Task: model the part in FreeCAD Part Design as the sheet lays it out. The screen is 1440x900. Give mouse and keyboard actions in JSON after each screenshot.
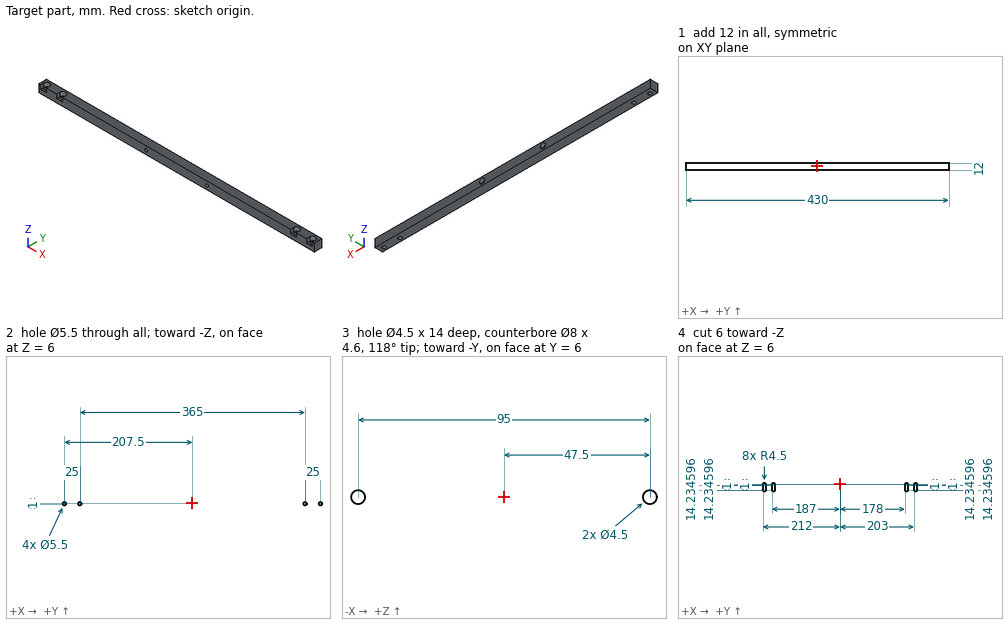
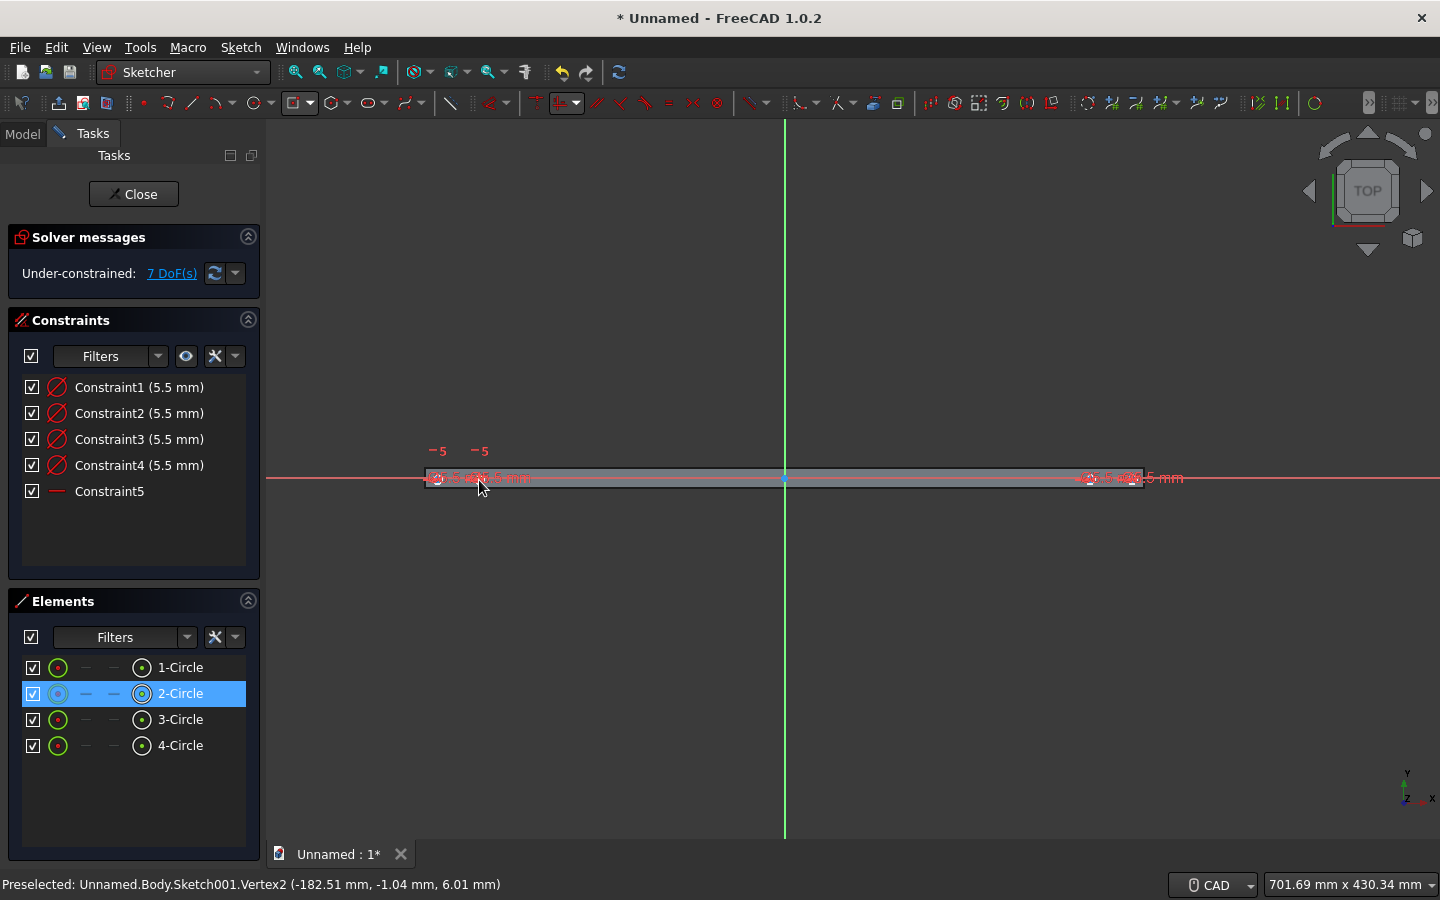
{"action": "left_click", "coordinate": [1090, 480]}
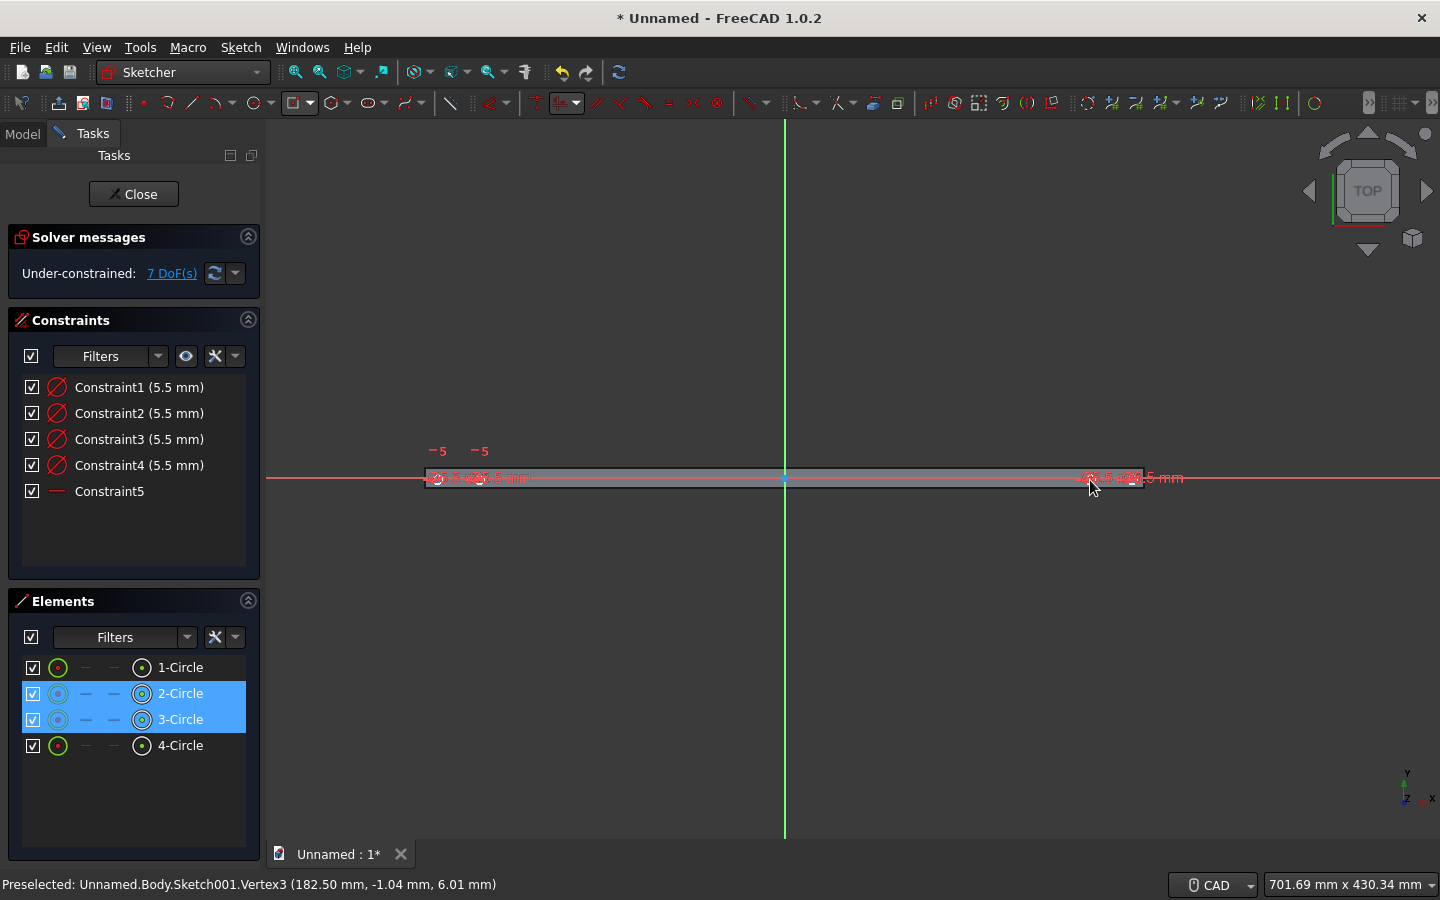
{"action": "left_click", "coordinate": [578, 104]}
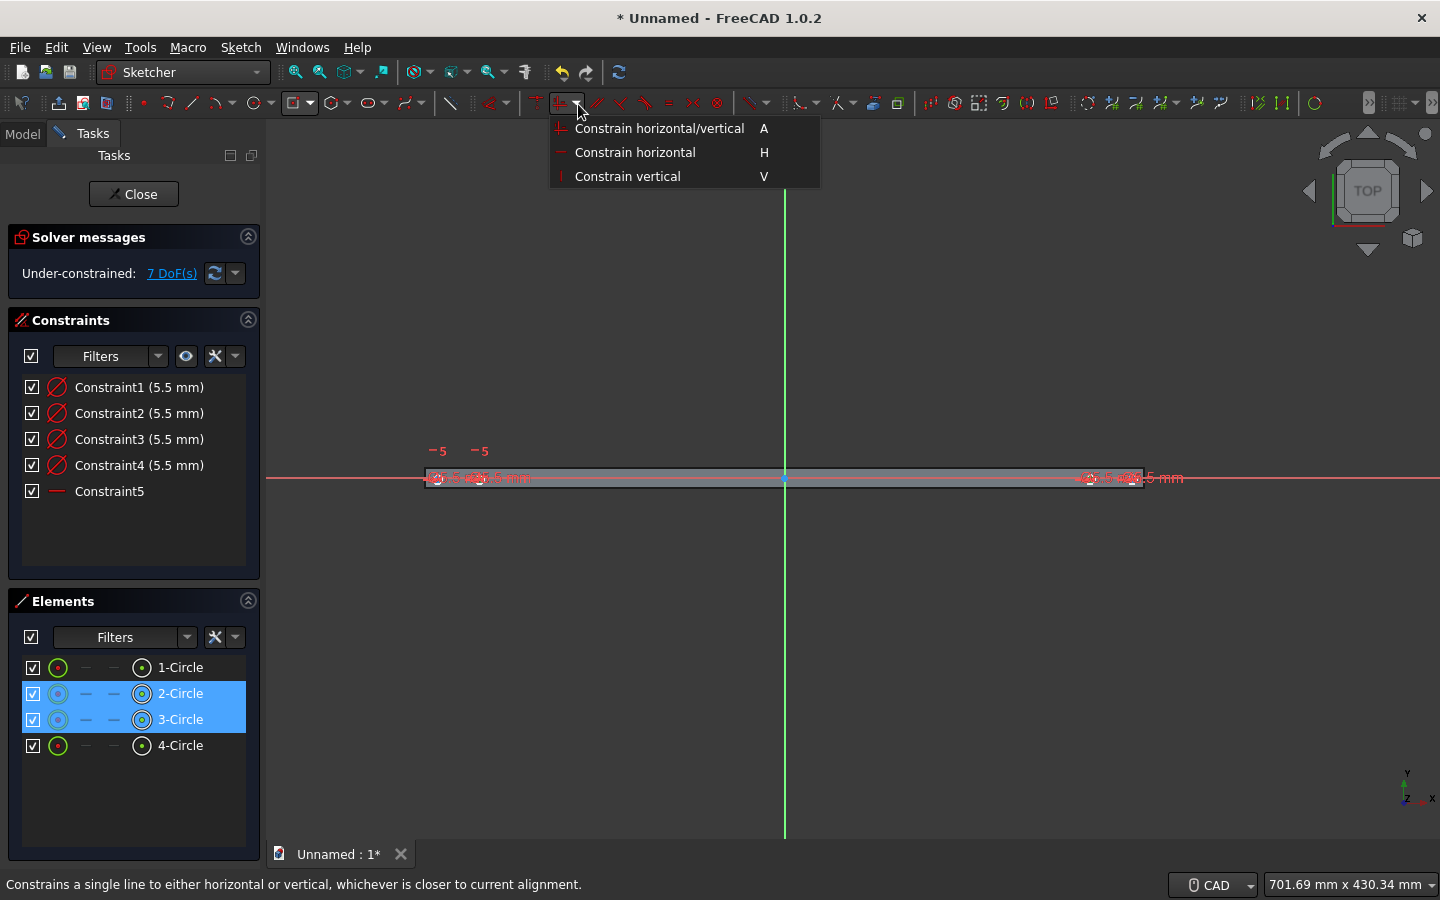
{"action": "left_click", "coordinate": [685, 152]}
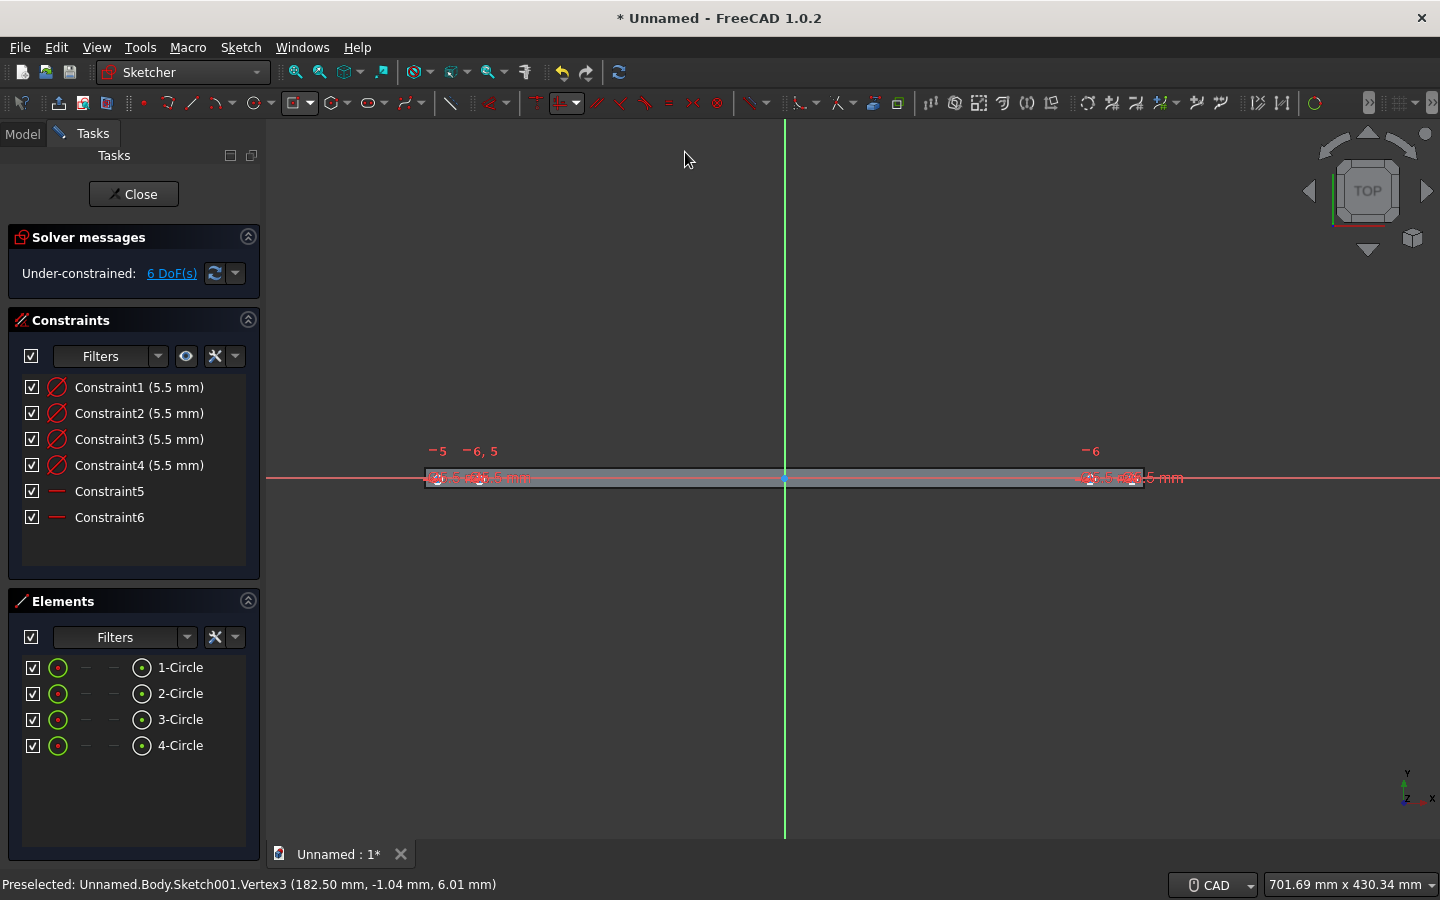
{"action": "left_click", "coordinate": [1090, 480]}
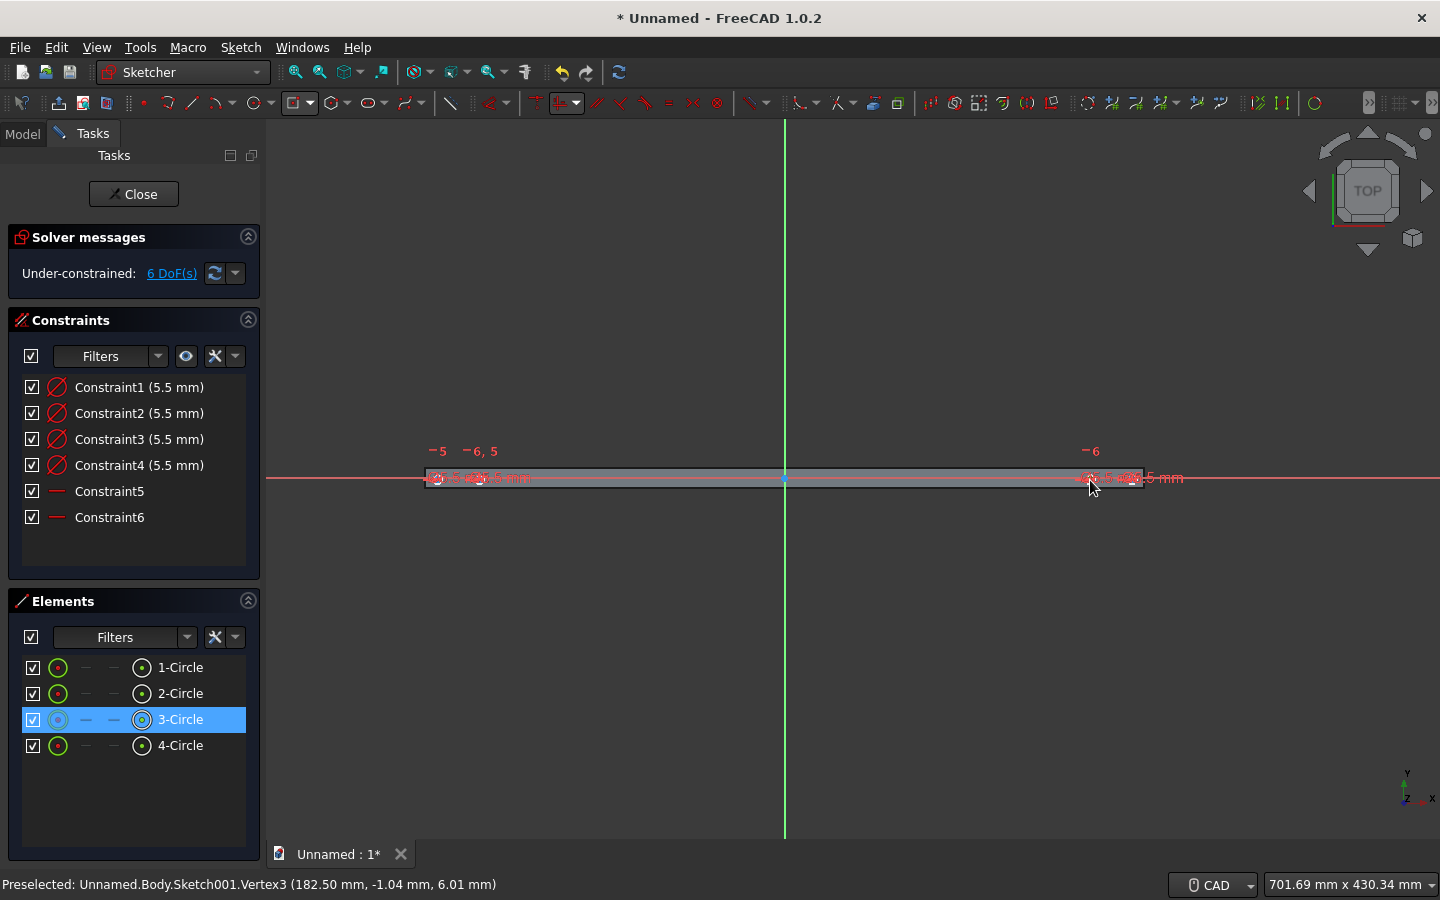
{"action": "left_click", "coordinate": [1132, 480]}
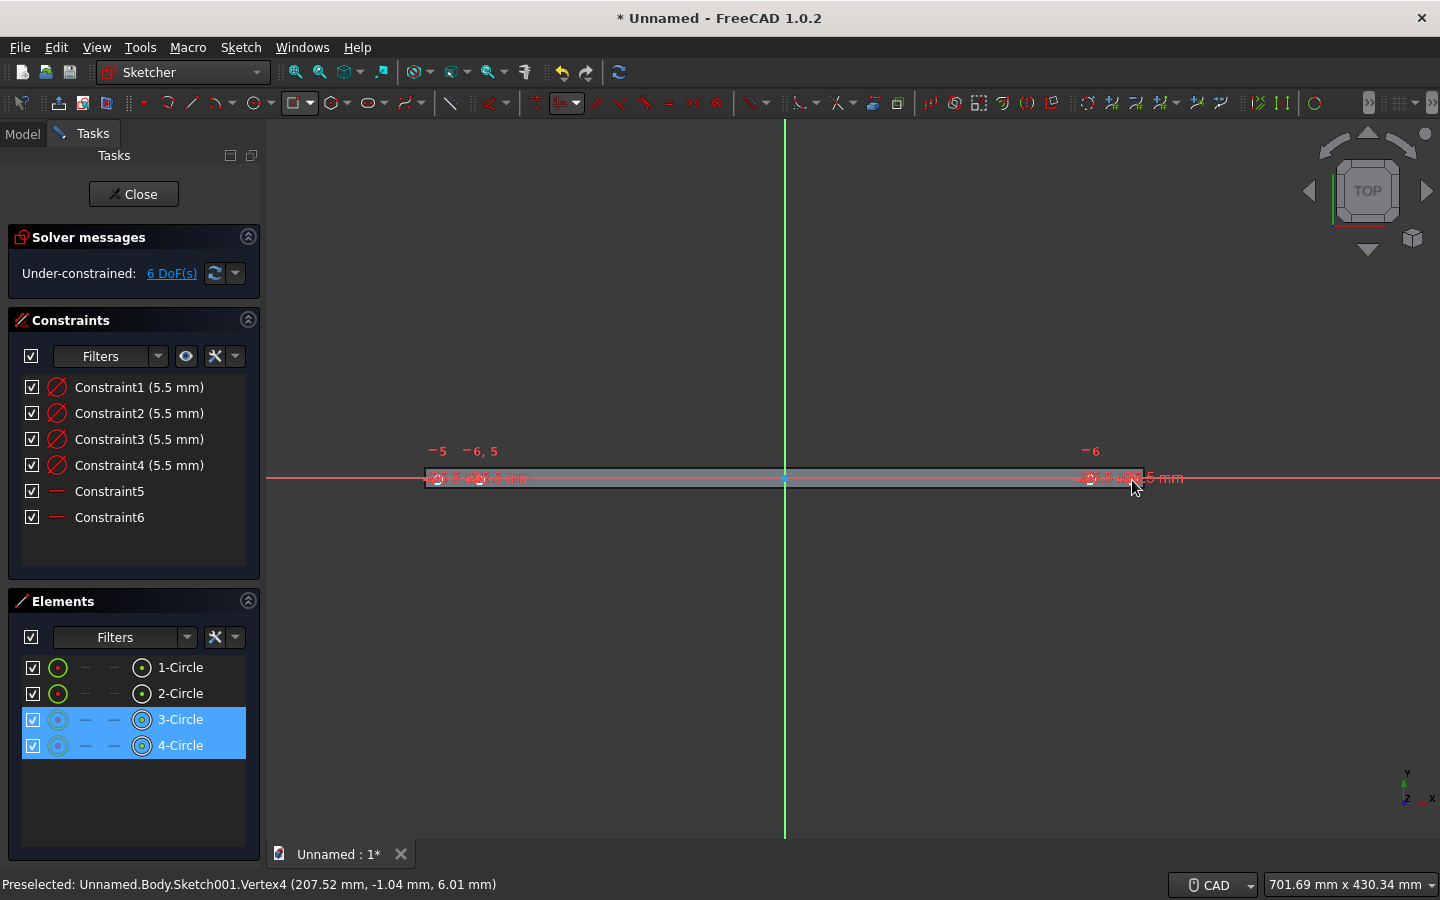
{"action": "key", "text": "h"}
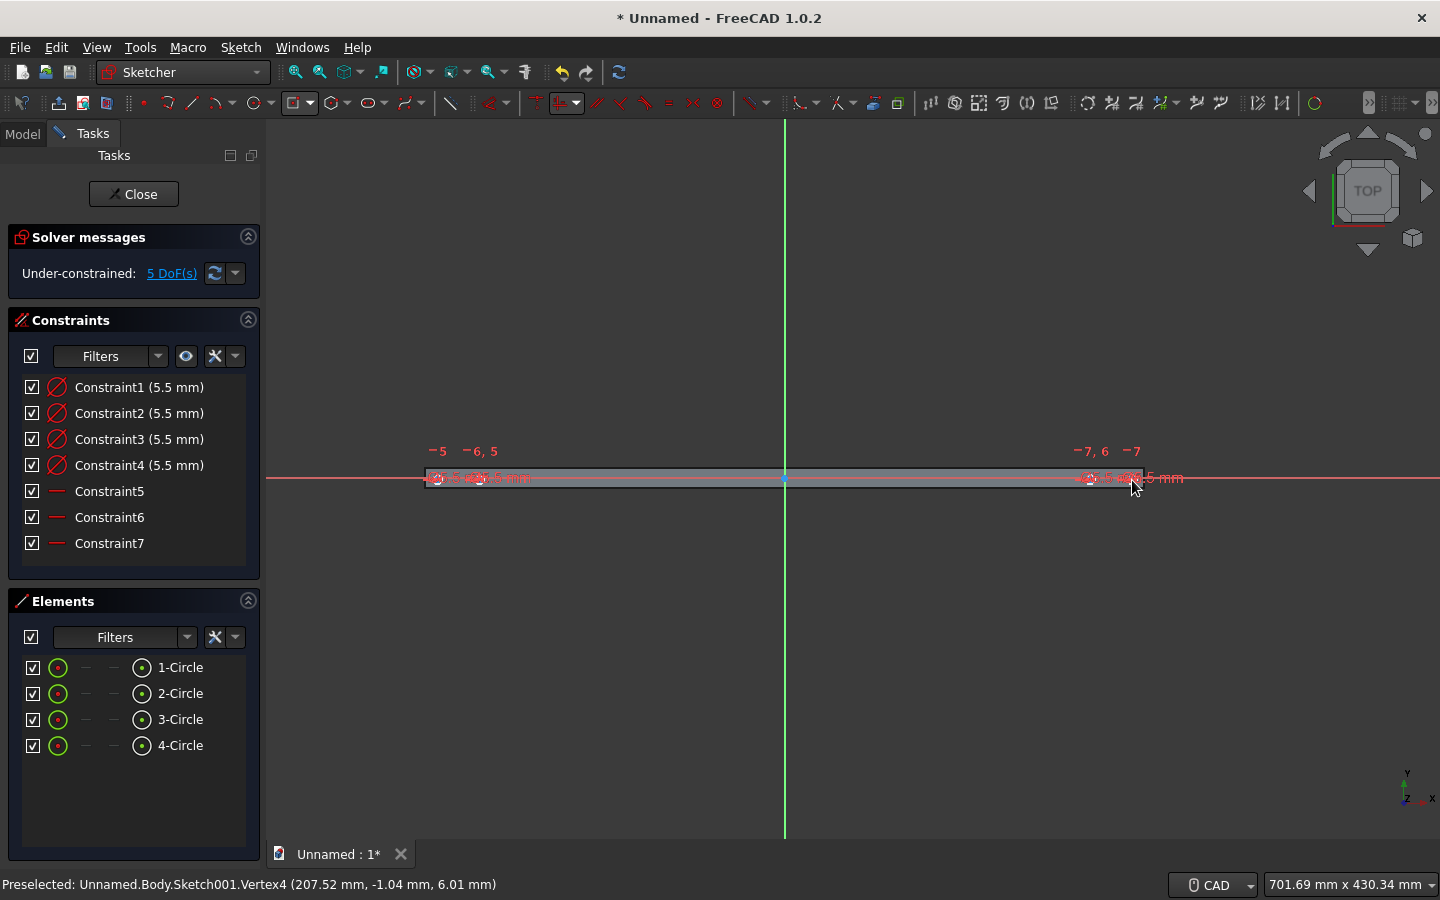
{"action": "left_click", "coordinate": [490, 104]}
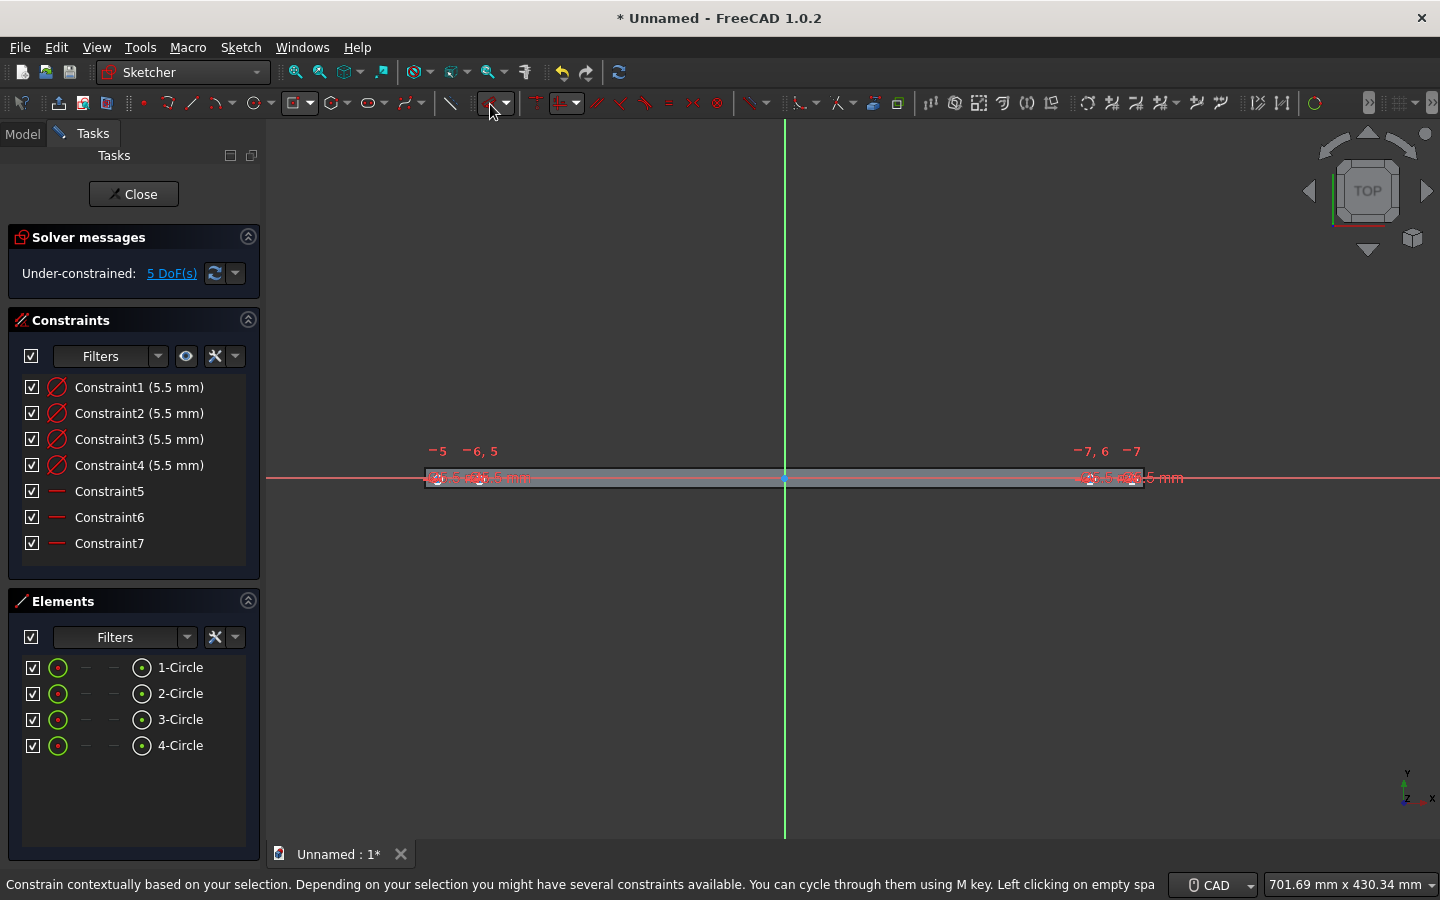
{"action": "scroll", "coordinate": [438, 480], "scroll_direction": "up", "scroll_amount": 16}